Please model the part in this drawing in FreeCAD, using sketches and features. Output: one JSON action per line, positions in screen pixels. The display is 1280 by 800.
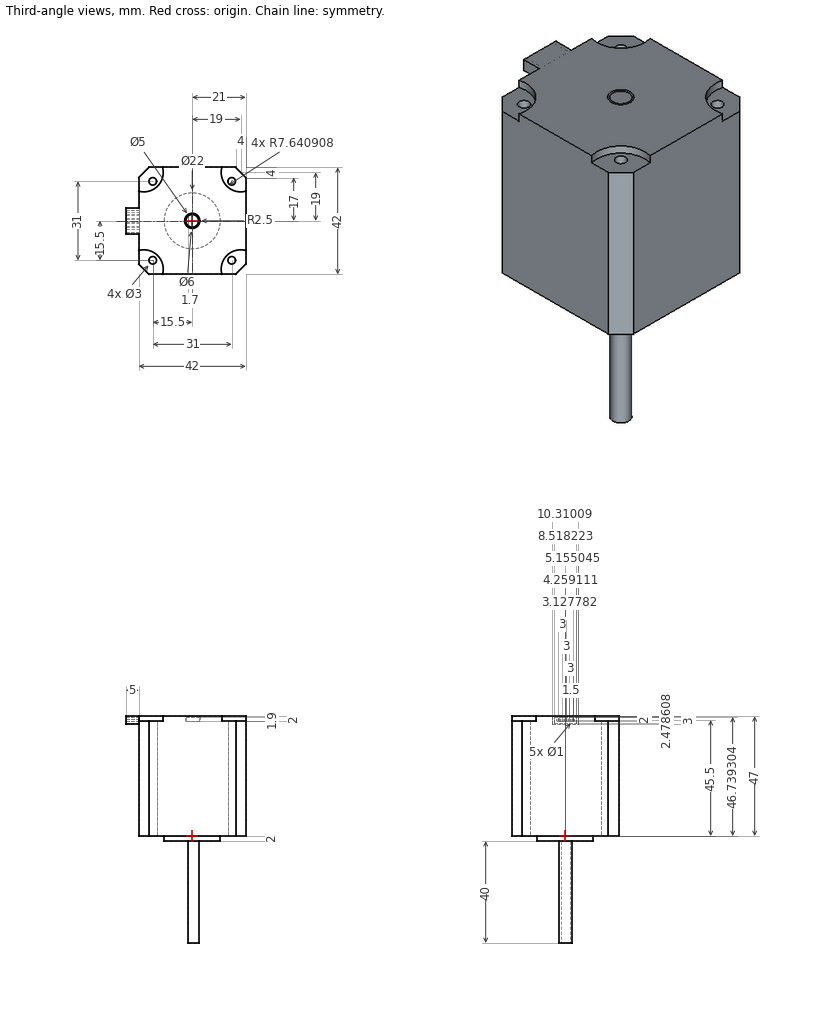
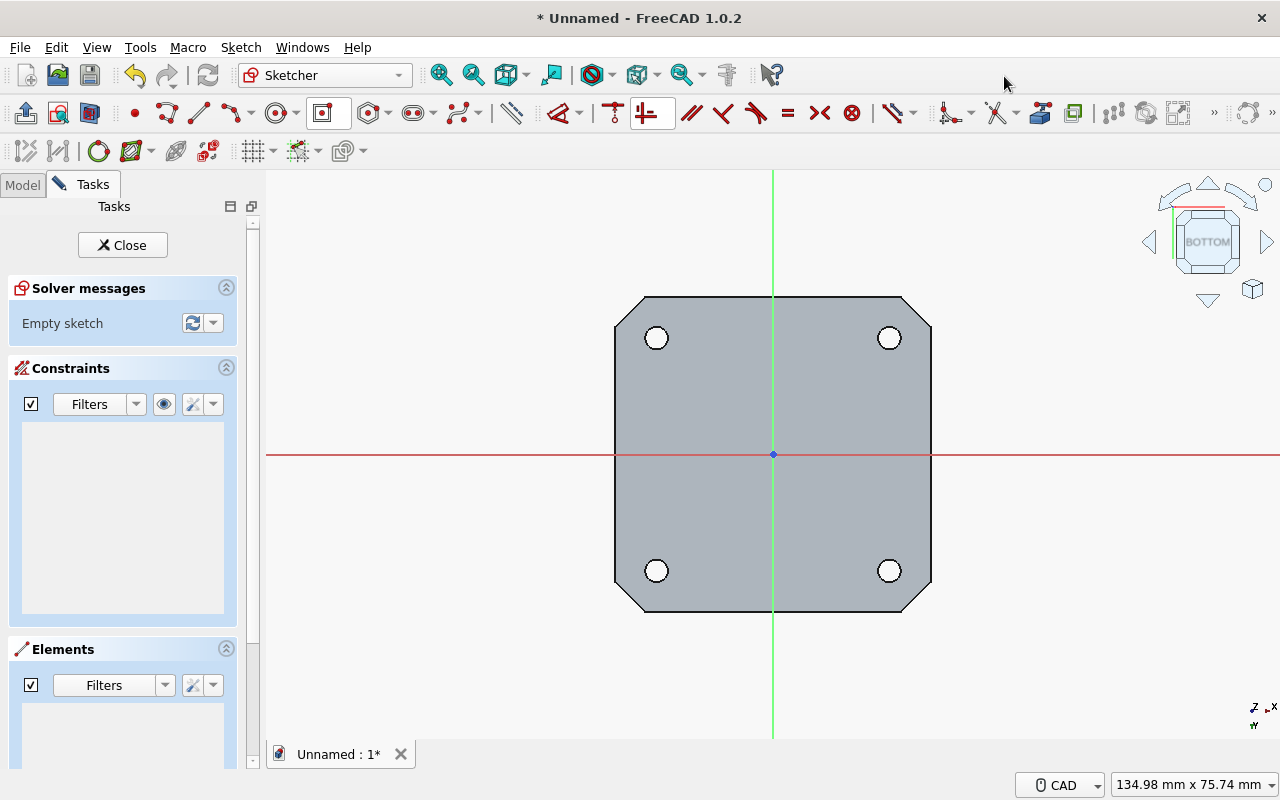
{"action": "scroll", "coordinate": [829, 455], "scroll_direction": "up", "scroll_amount": 4}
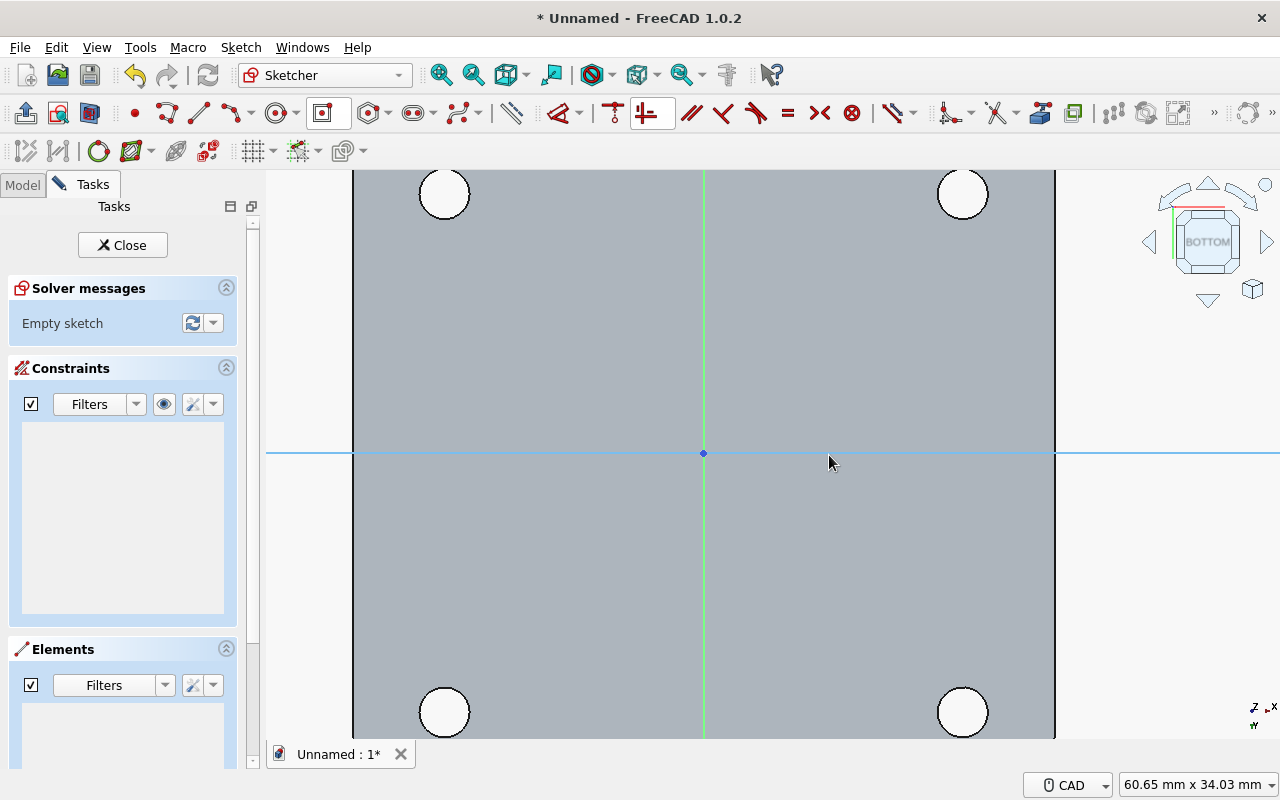
{"action": "left_click", "coordinate": [276, 114]}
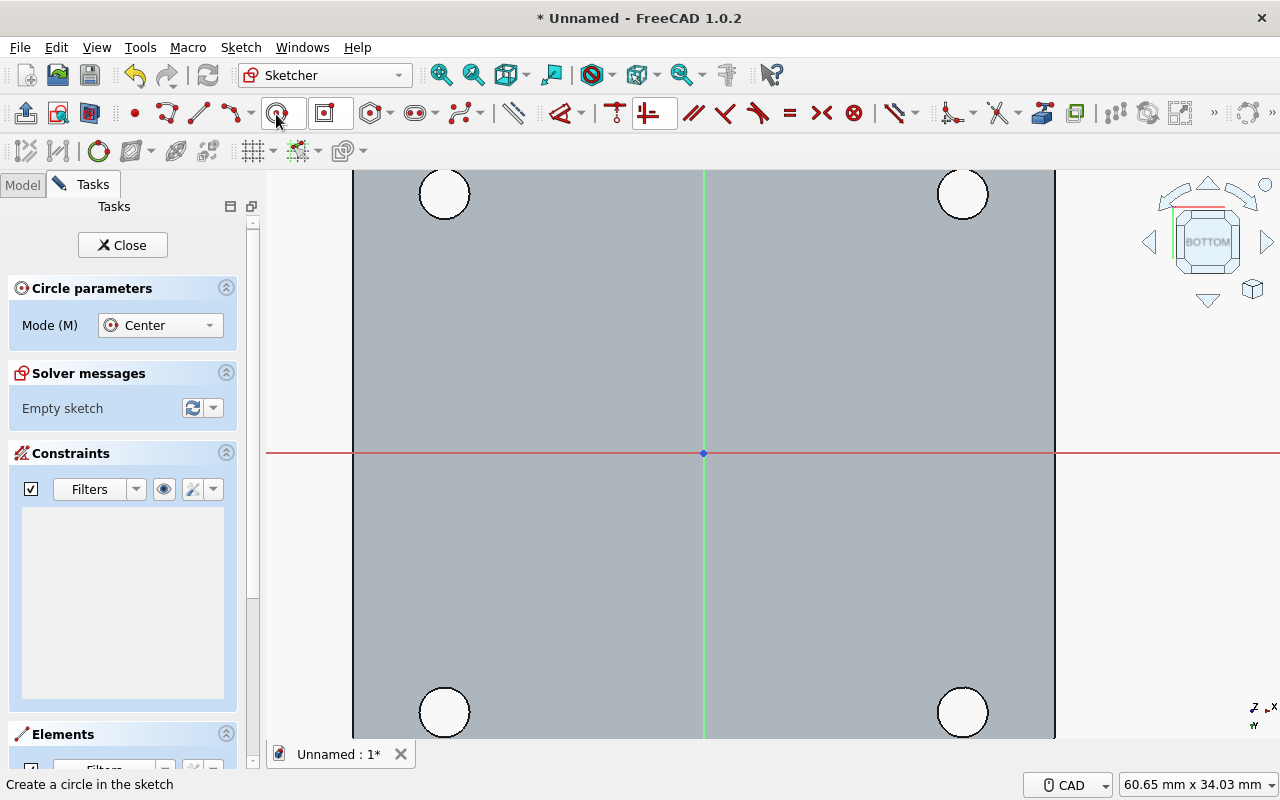
{"action": "left_click", "coordinate": [704, 453]}
{"action": "left_click", "coordinate": [834, 323]}
{"action": "key", "text": "Escape"}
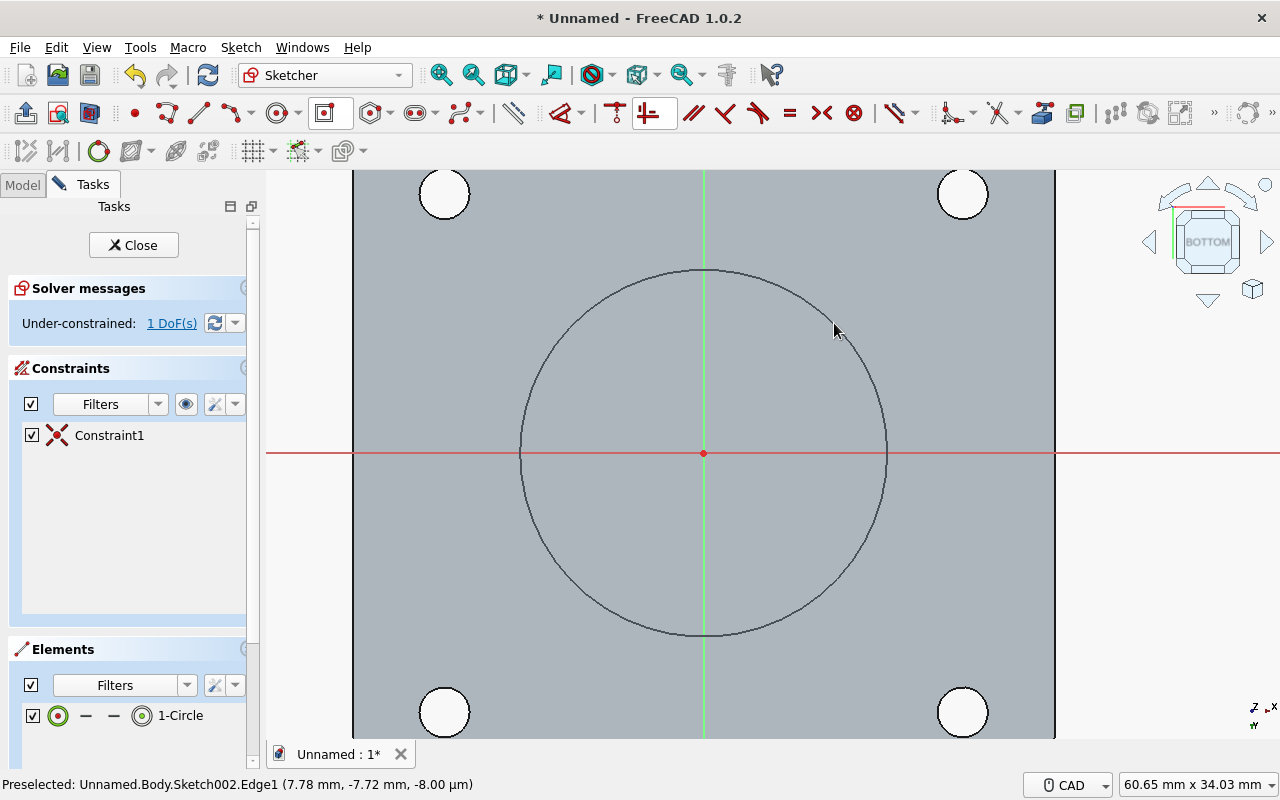
{"action": "left_click", "coordinate": [560, 114]}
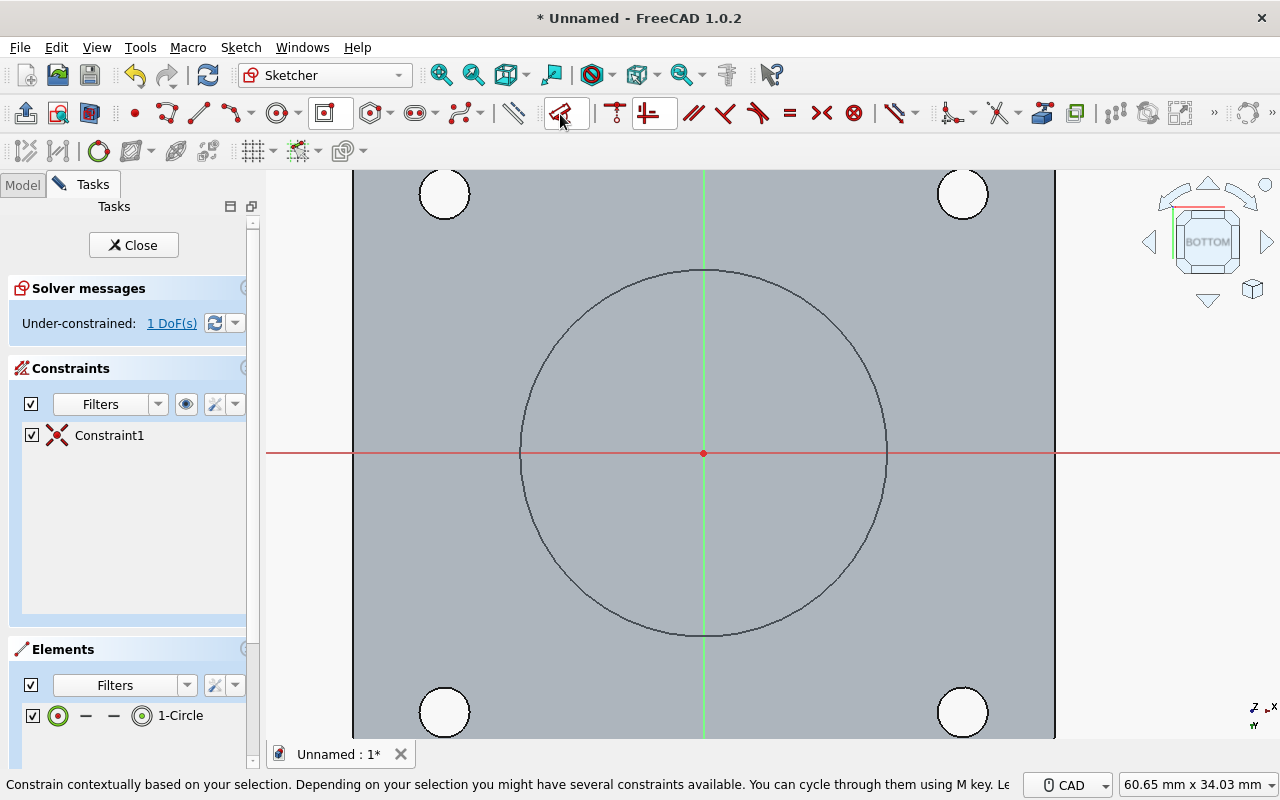
{"action": "left_click", "coordinate": [833, 323]}
{"action": "left_click", "coordinate": [856, 300]}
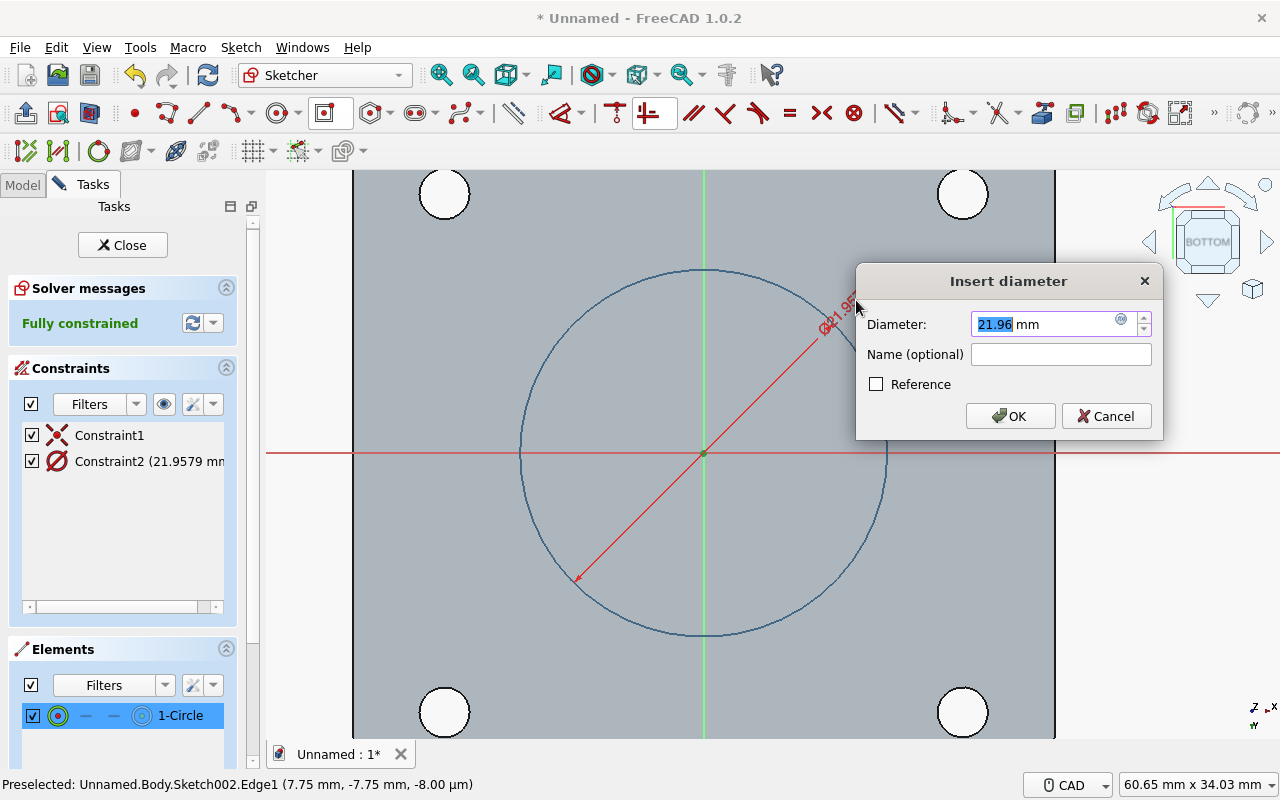
{"action": "type", "text": "22"}
{"action": "key", "text": "Return"}
{"action": "key", "text": "Escape"}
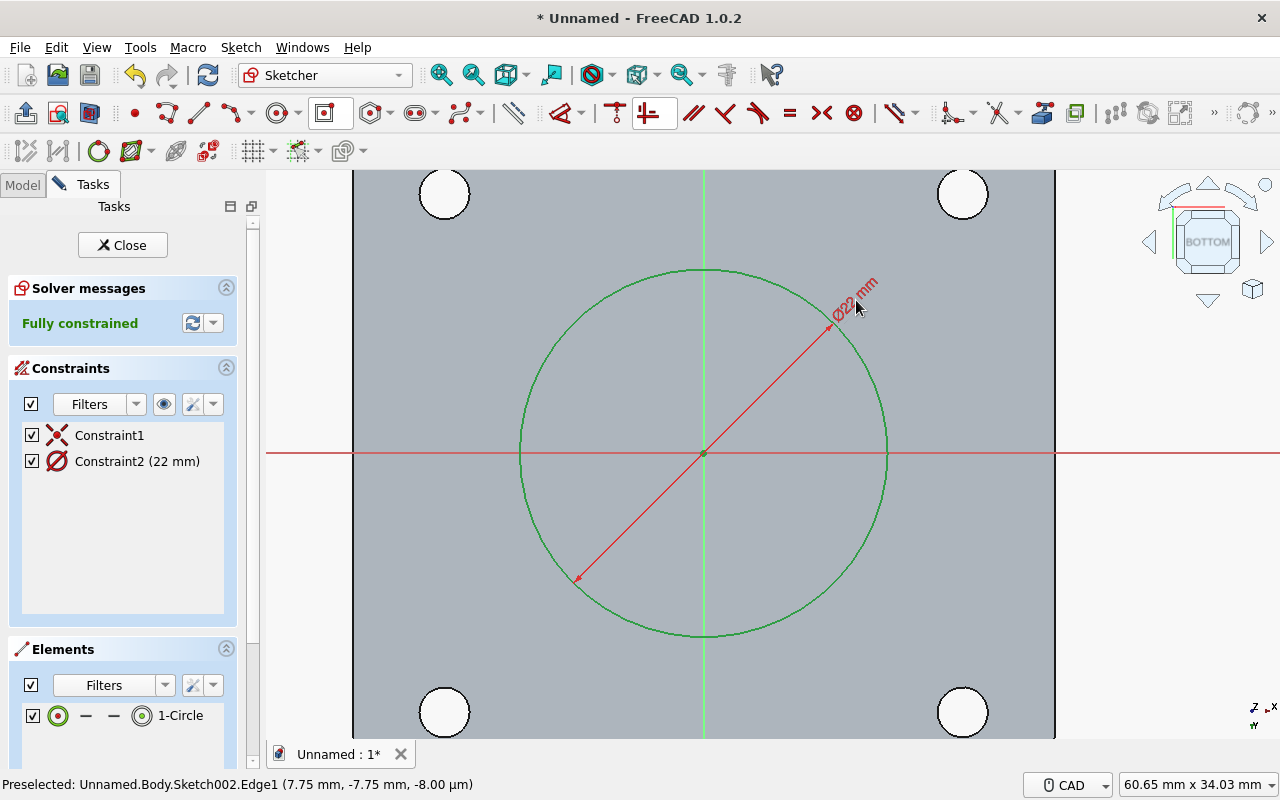
{"action": "left_click", "coordinate": [123, 245]}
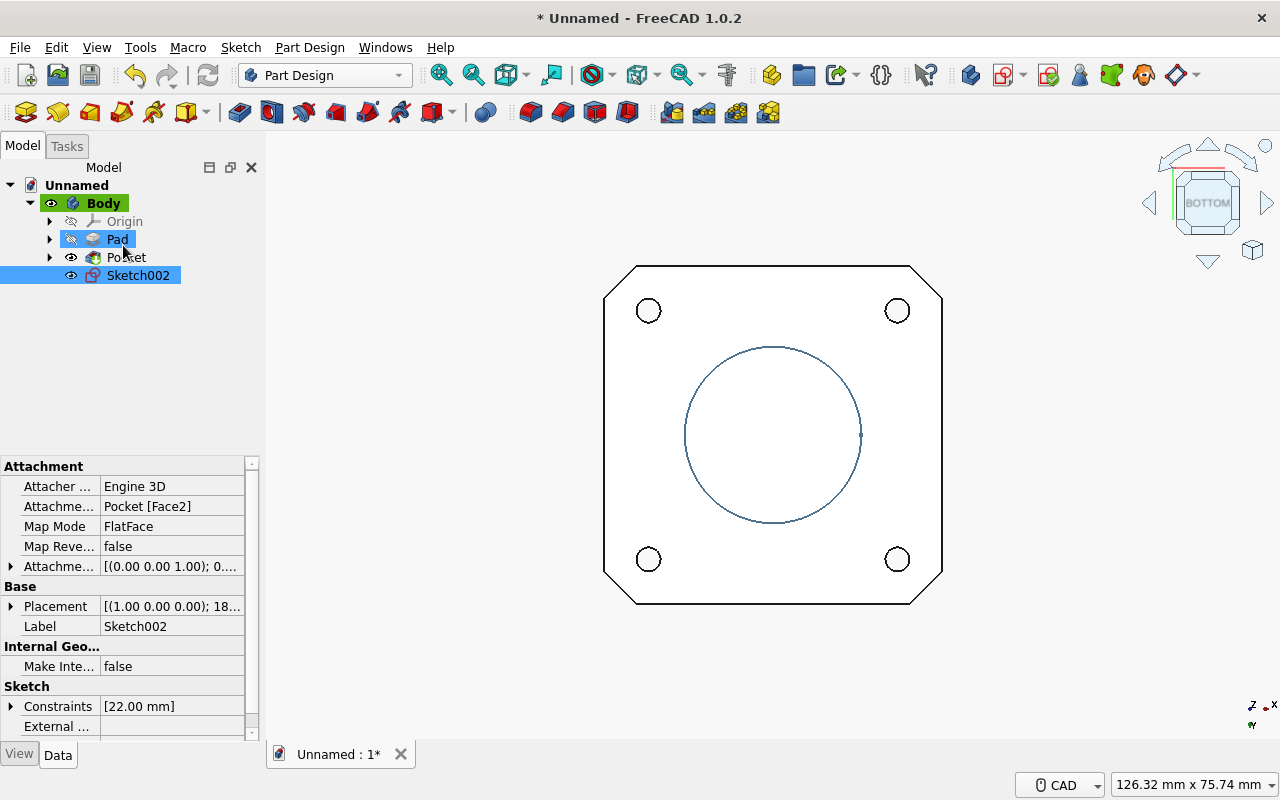
{"action": "left_click", "coordinate": [26, 112]}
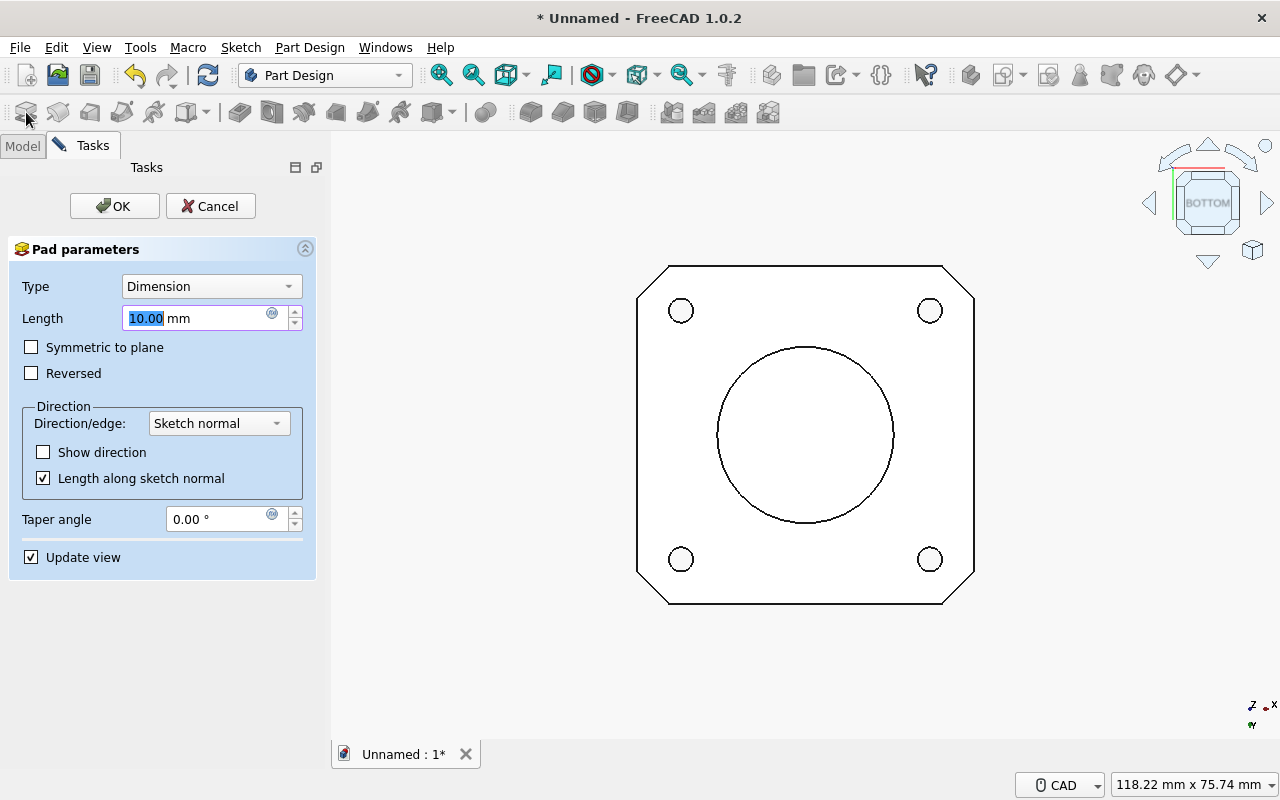
{"action": "type", "text": "2"}
{"action": "key", "text": "Tab"}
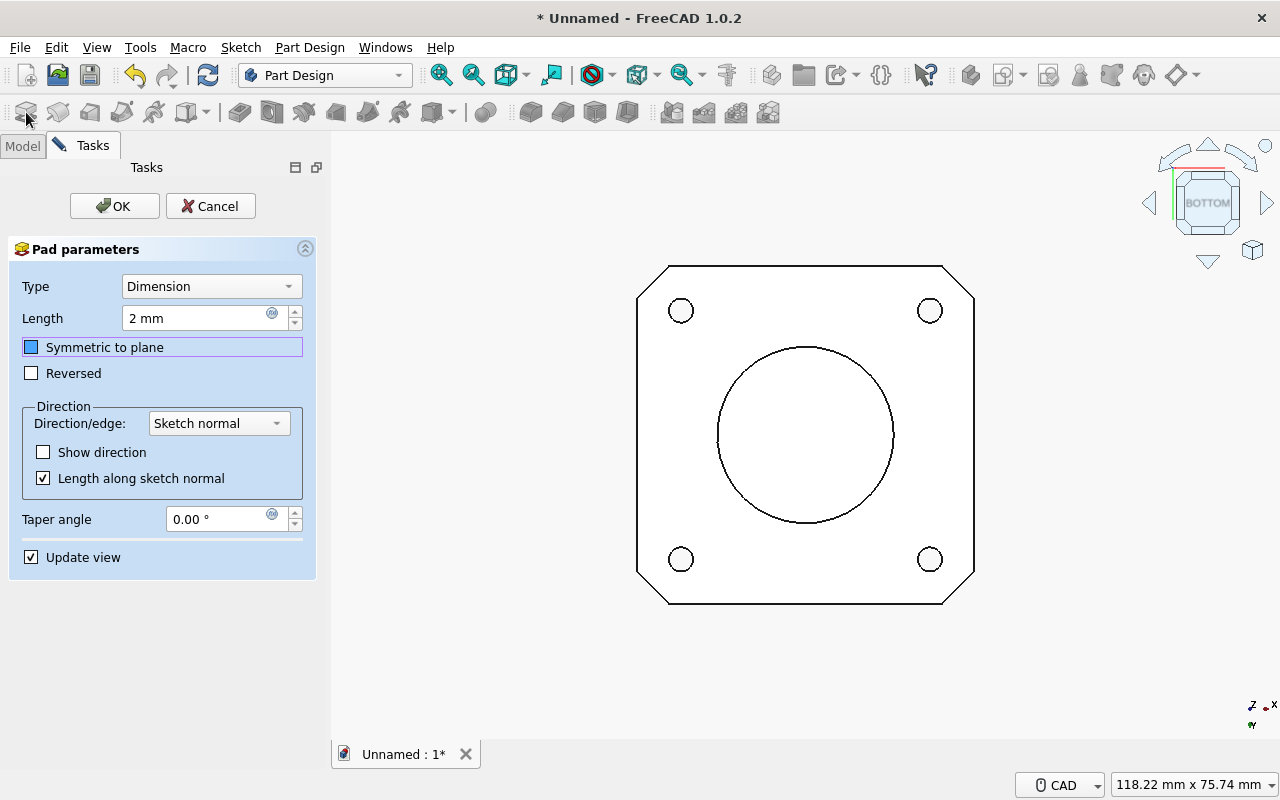
{"action": "left_click", "coordinate": [115, 206]}